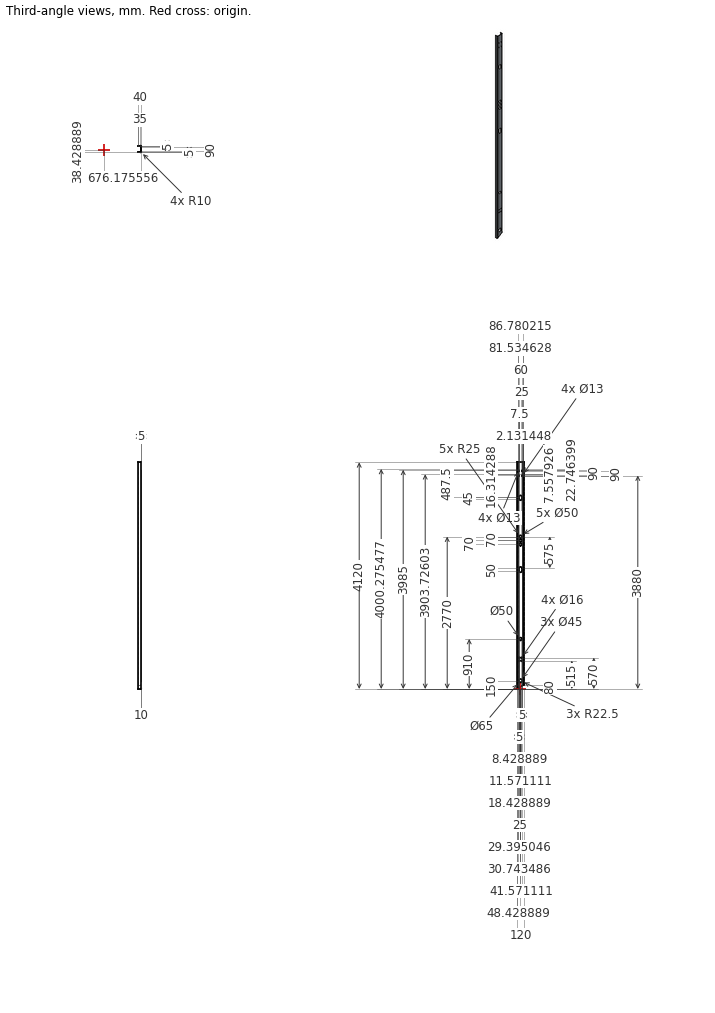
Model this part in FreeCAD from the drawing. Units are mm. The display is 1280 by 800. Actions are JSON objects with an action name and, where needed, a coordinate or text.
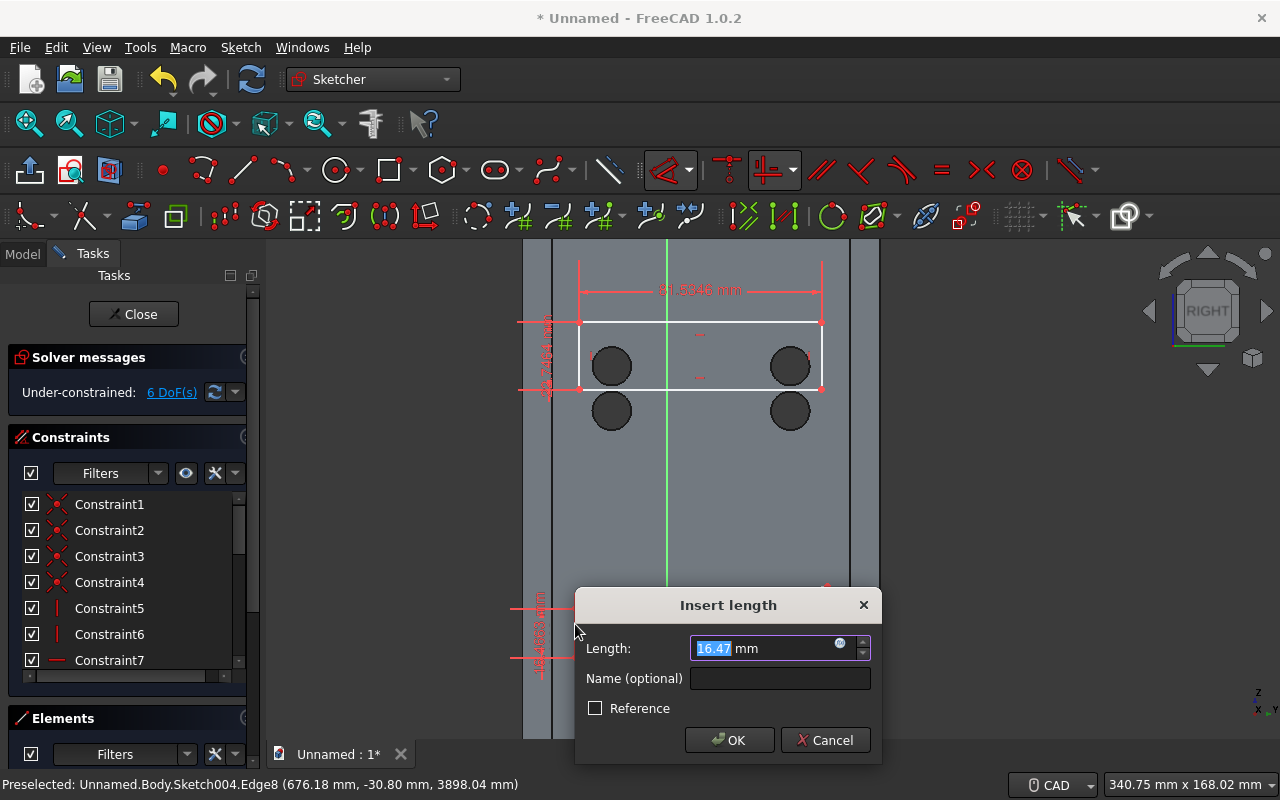
{"action": "type", "text": "16.314288"}
{"action": "key", "text": "Return"}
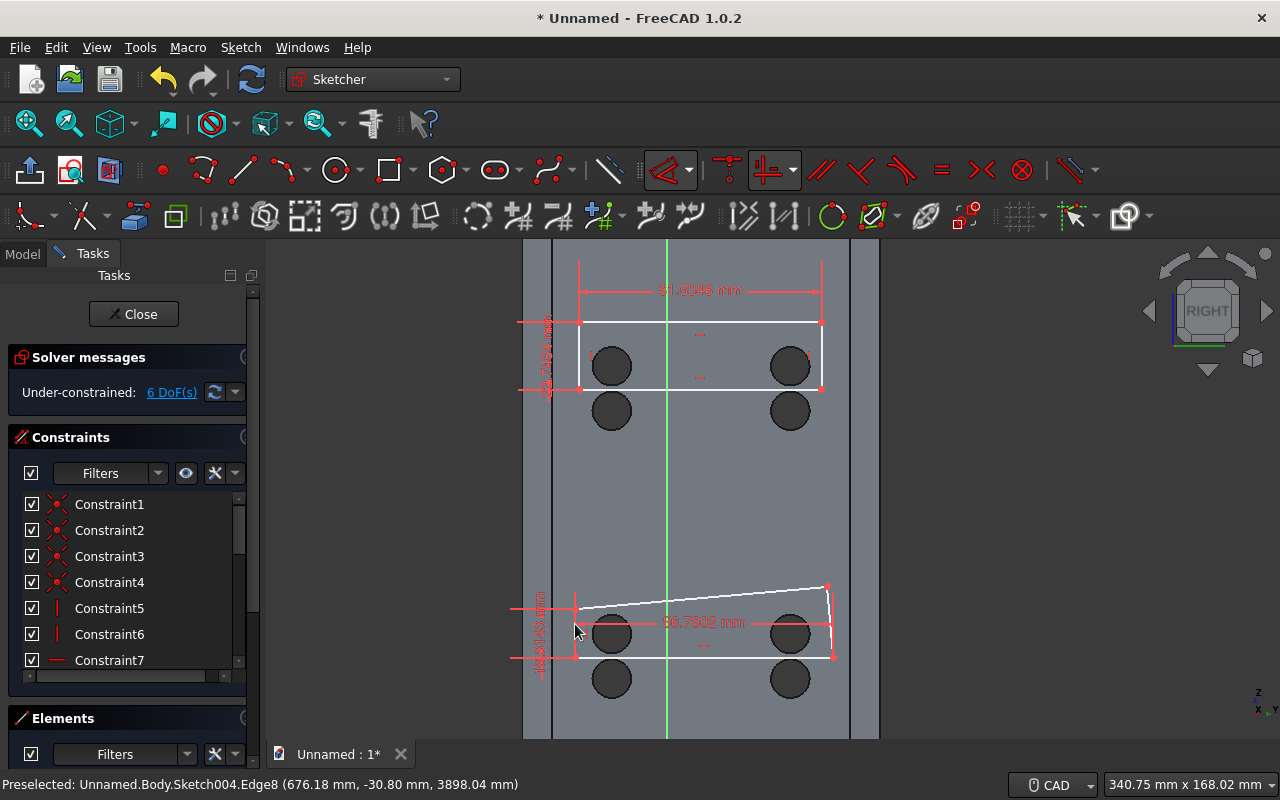
{"action": "scroll", "coordinate": [831, 637], "scroll_direction": "up", "scroll_amount": 10}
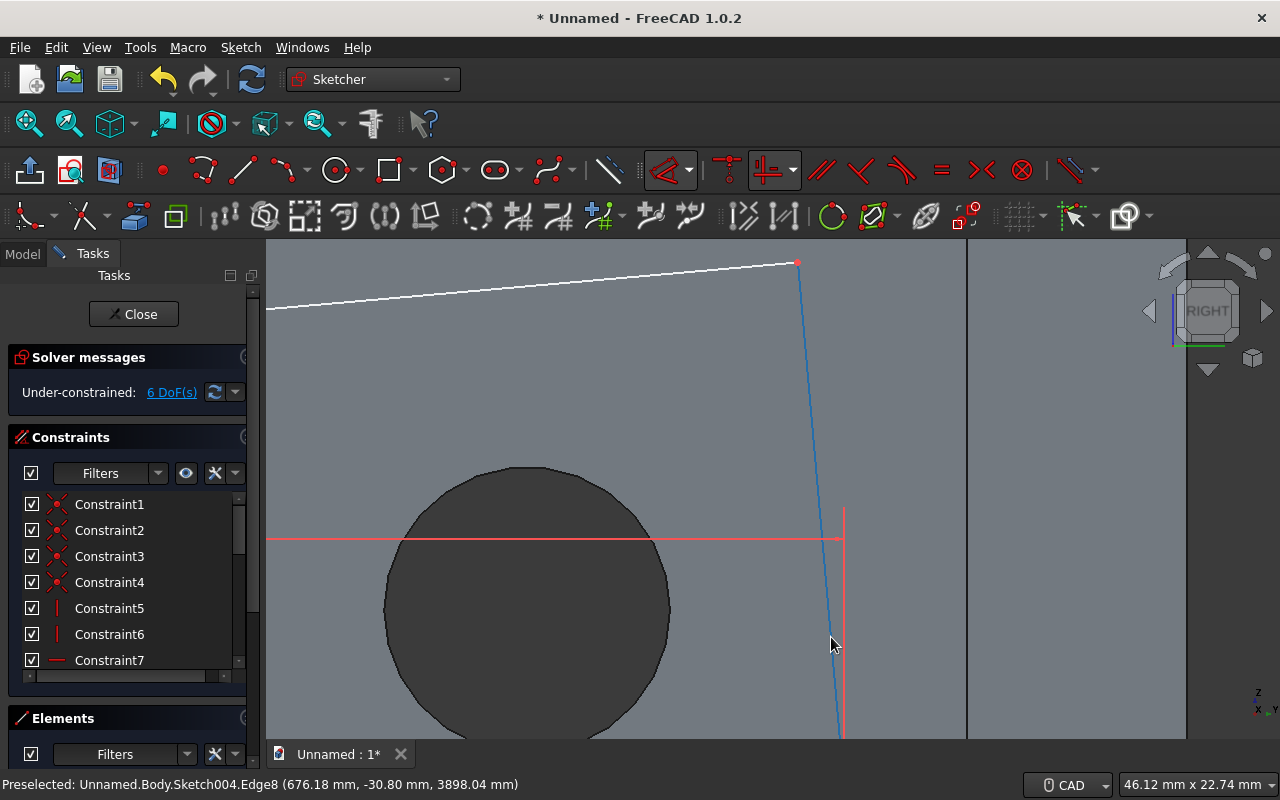
{"action": "left_click", "coordinate": [830, 628]}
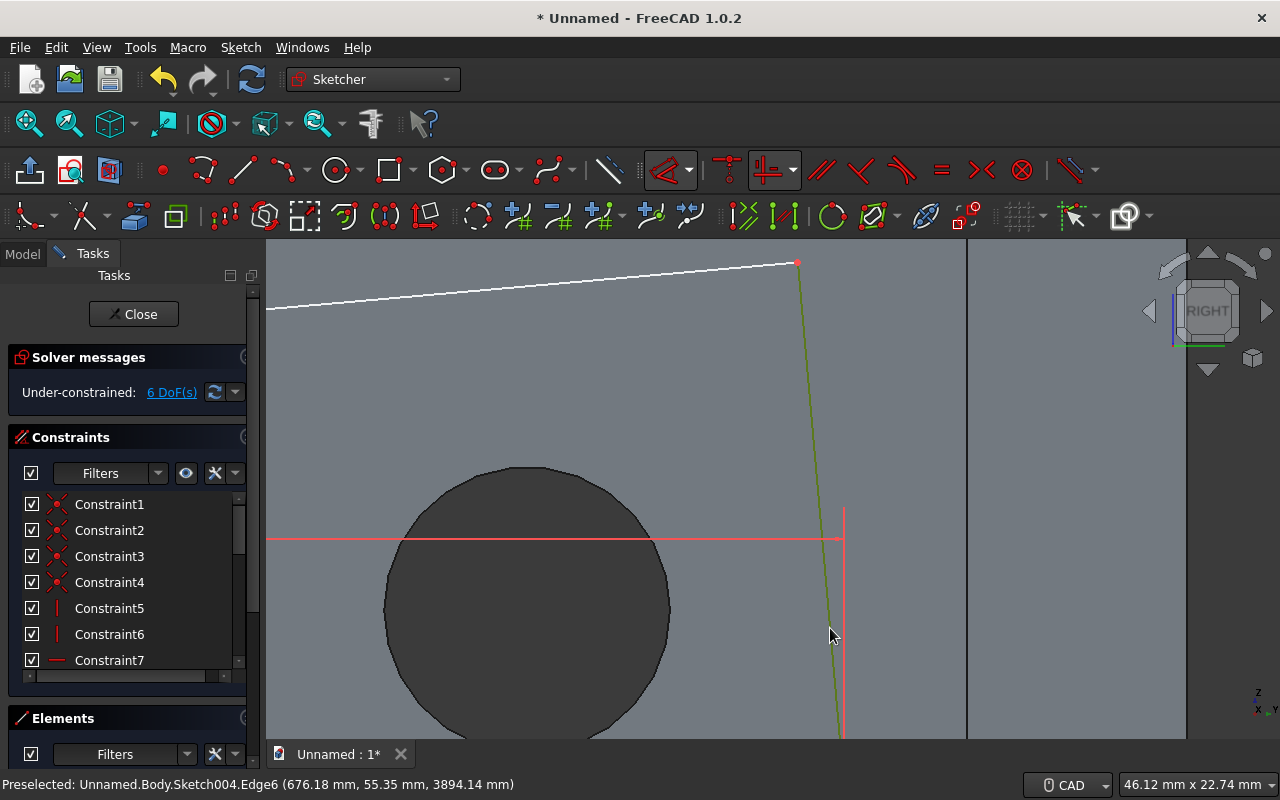
{"action": "key", "text": "l"}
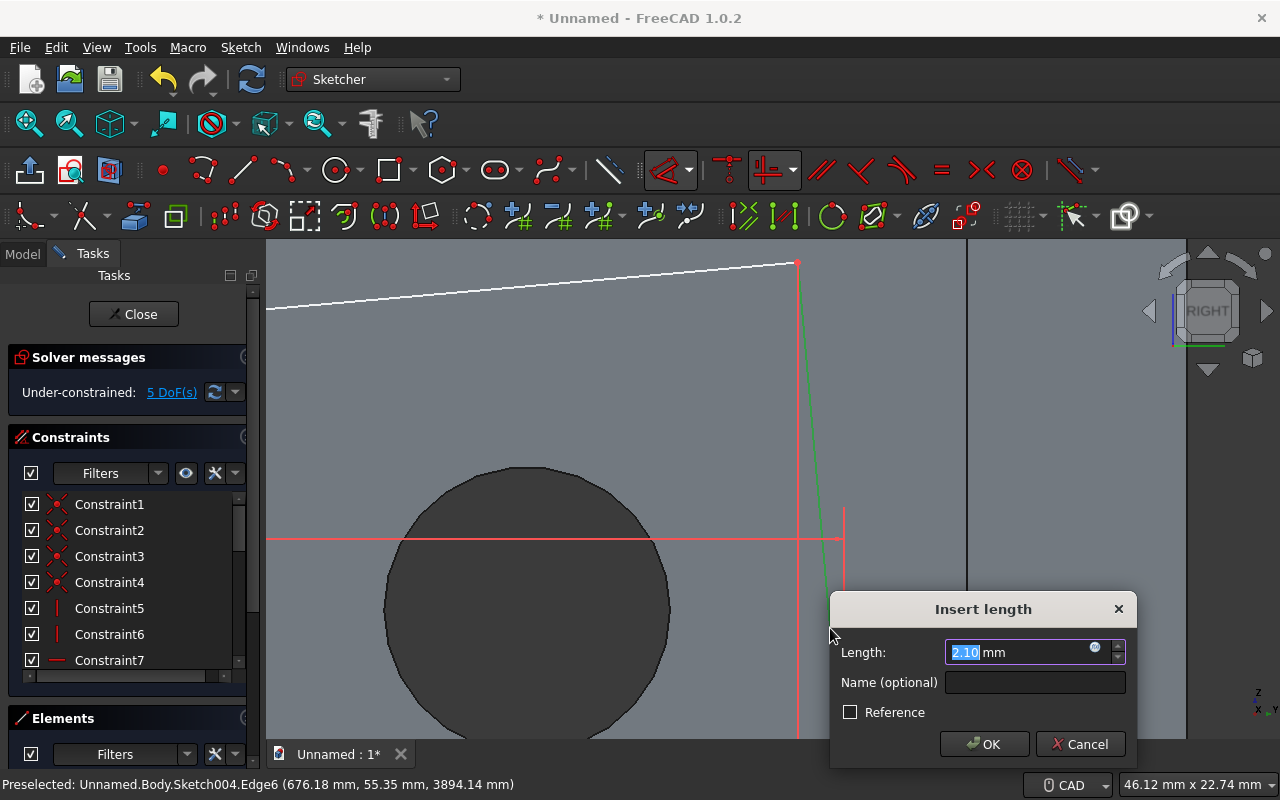
{"action": "type", "text": "2.131448"}
{"action": "key", "text": "Return"}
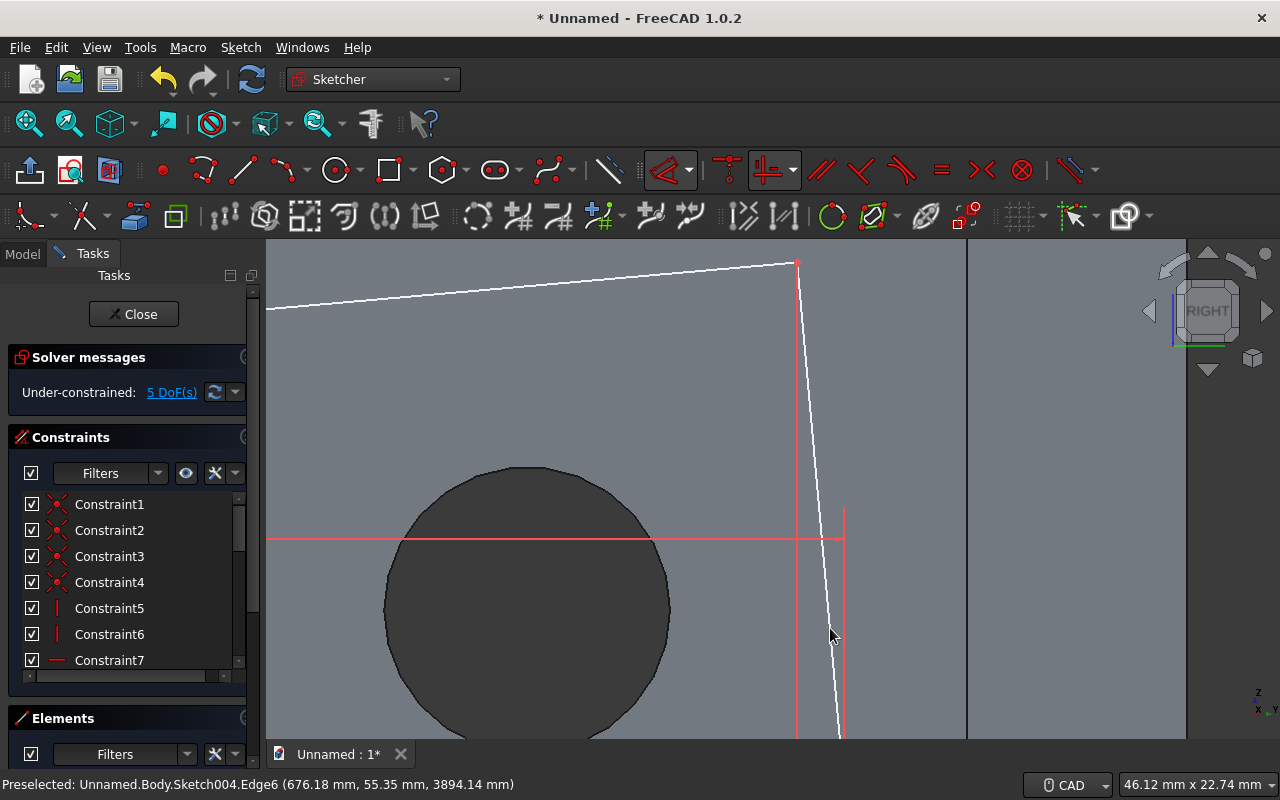
{"action": "scroll", "coordinate": [832, 638], "scroll_direction": "down", "scroll_amount": 10}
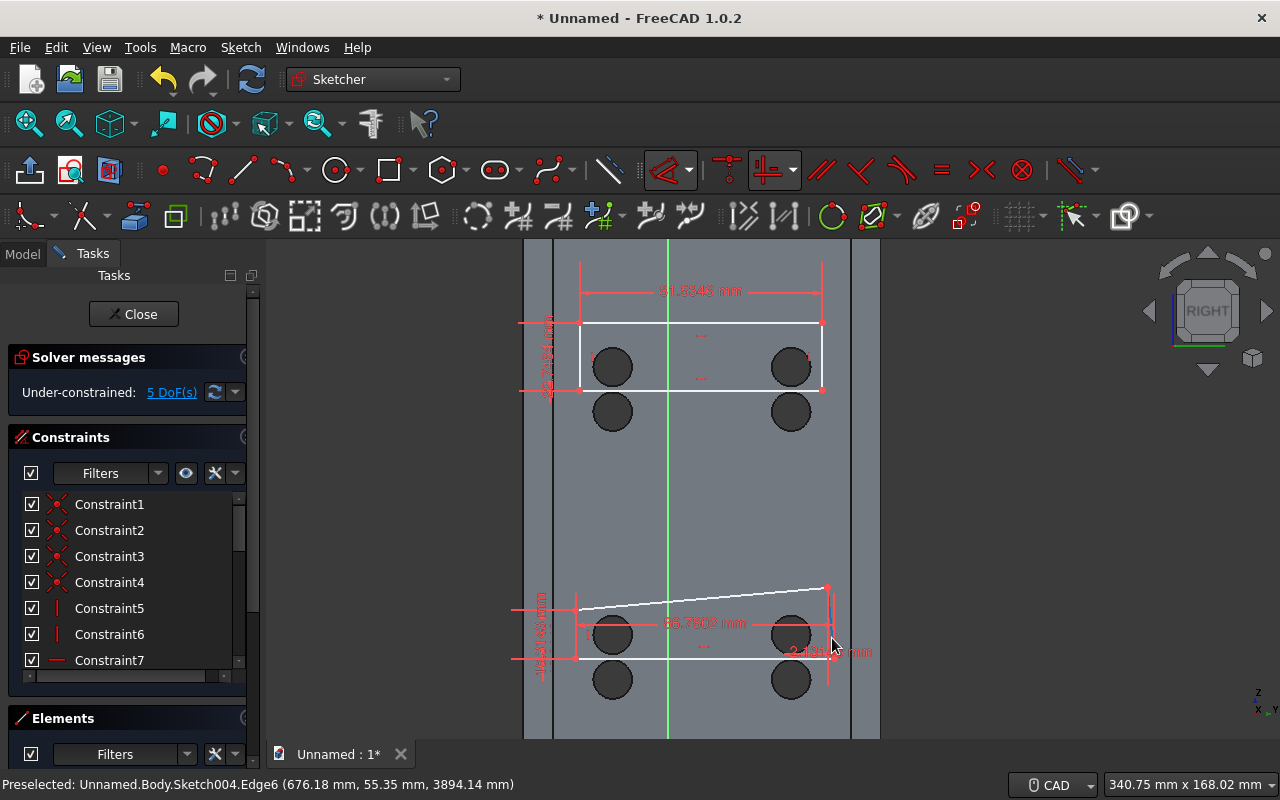
{"action": "scroll", "coordinate": [777, 592], "scroll_direction": "up", "scroll_amount": 3}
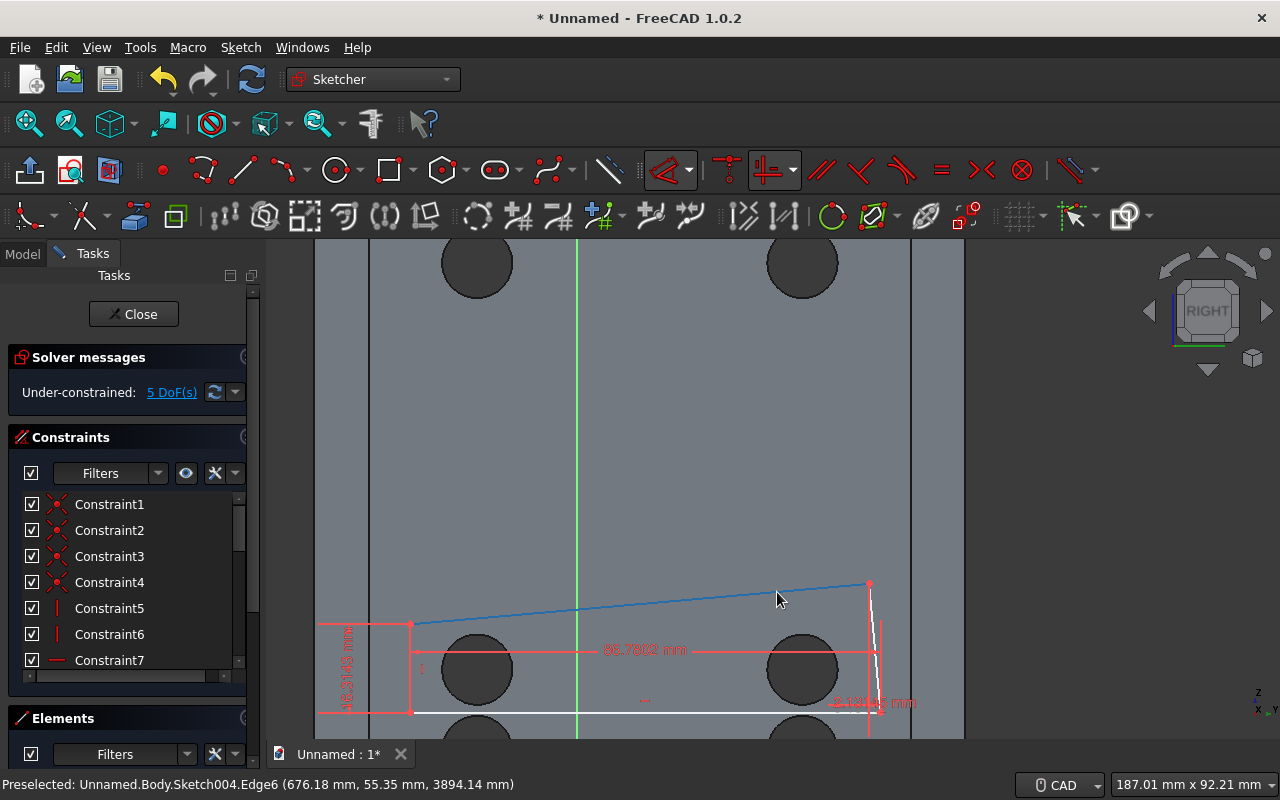
{"action": "left_click", "coordinate": [777, 592]}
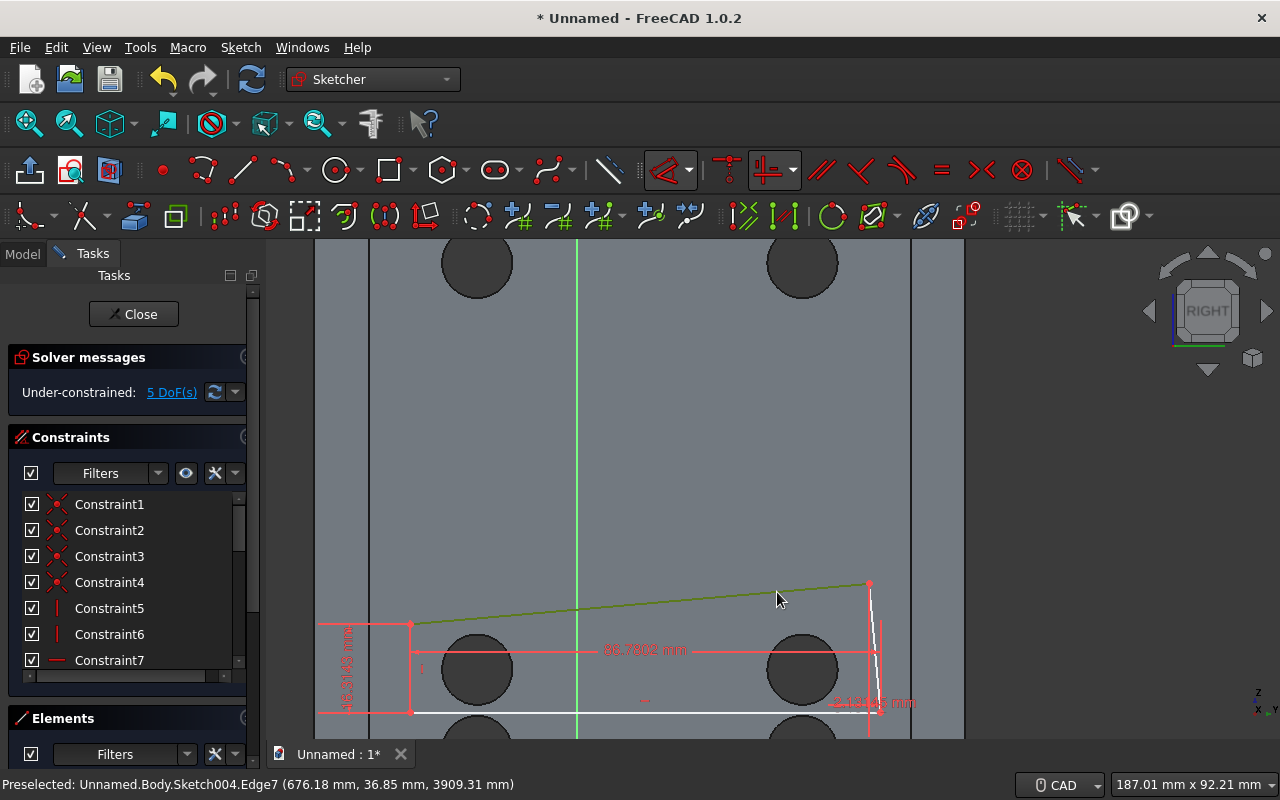
{"action": "key", "text": "i"}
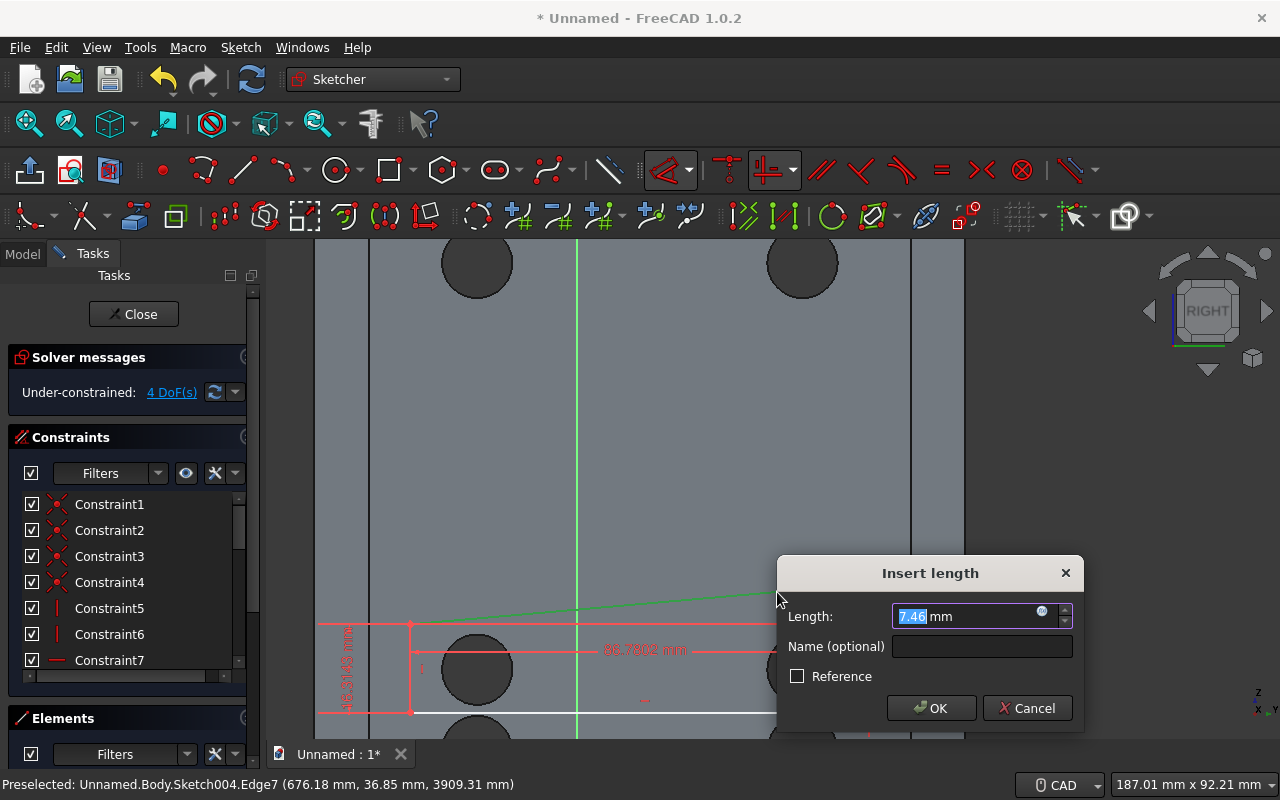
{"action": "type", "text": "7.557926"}
{"action": "key", "text": "Return"}